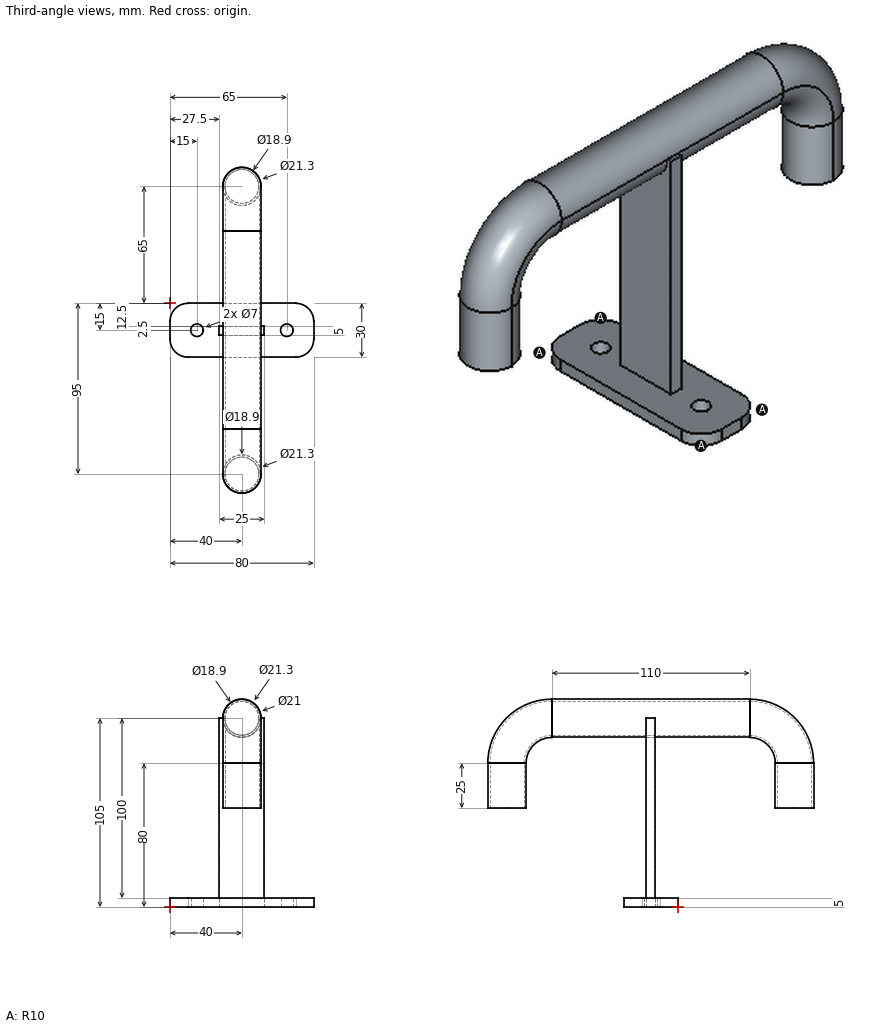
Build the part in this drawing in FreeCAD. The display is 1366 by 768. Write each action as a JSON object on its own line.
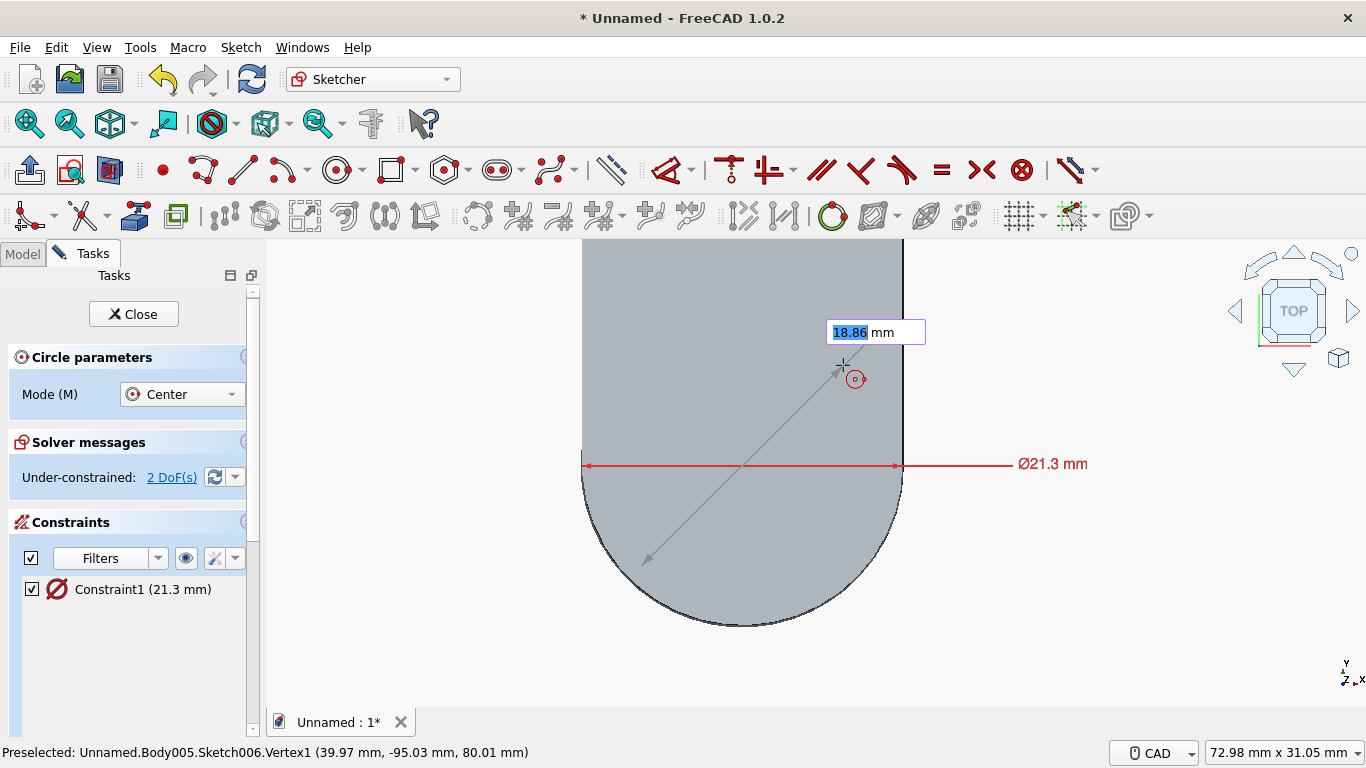
{"action": "type", "text": "18.9"}
{"action": "key", "text": "Return"}
{"action": "key", "text": "Escape"}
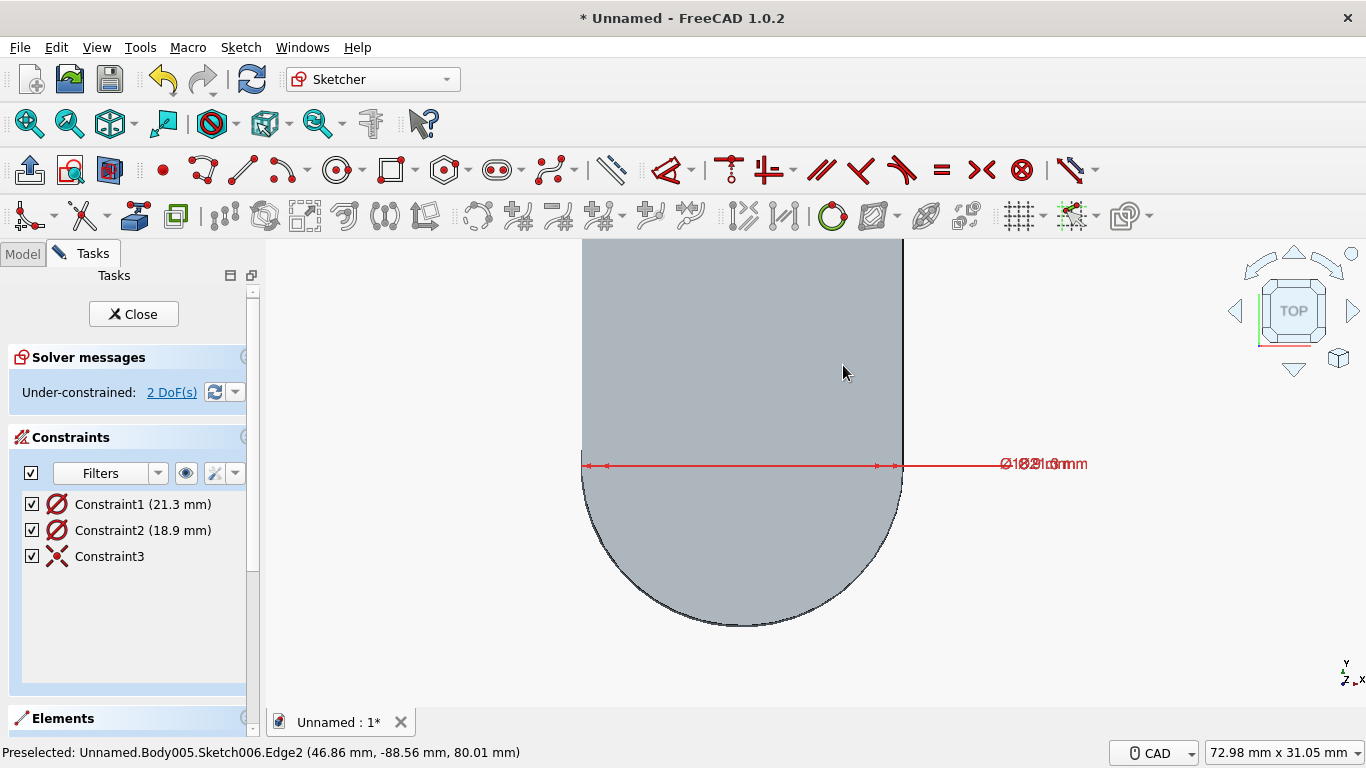
{"action": "left_click", "coordinate": [666, 170]}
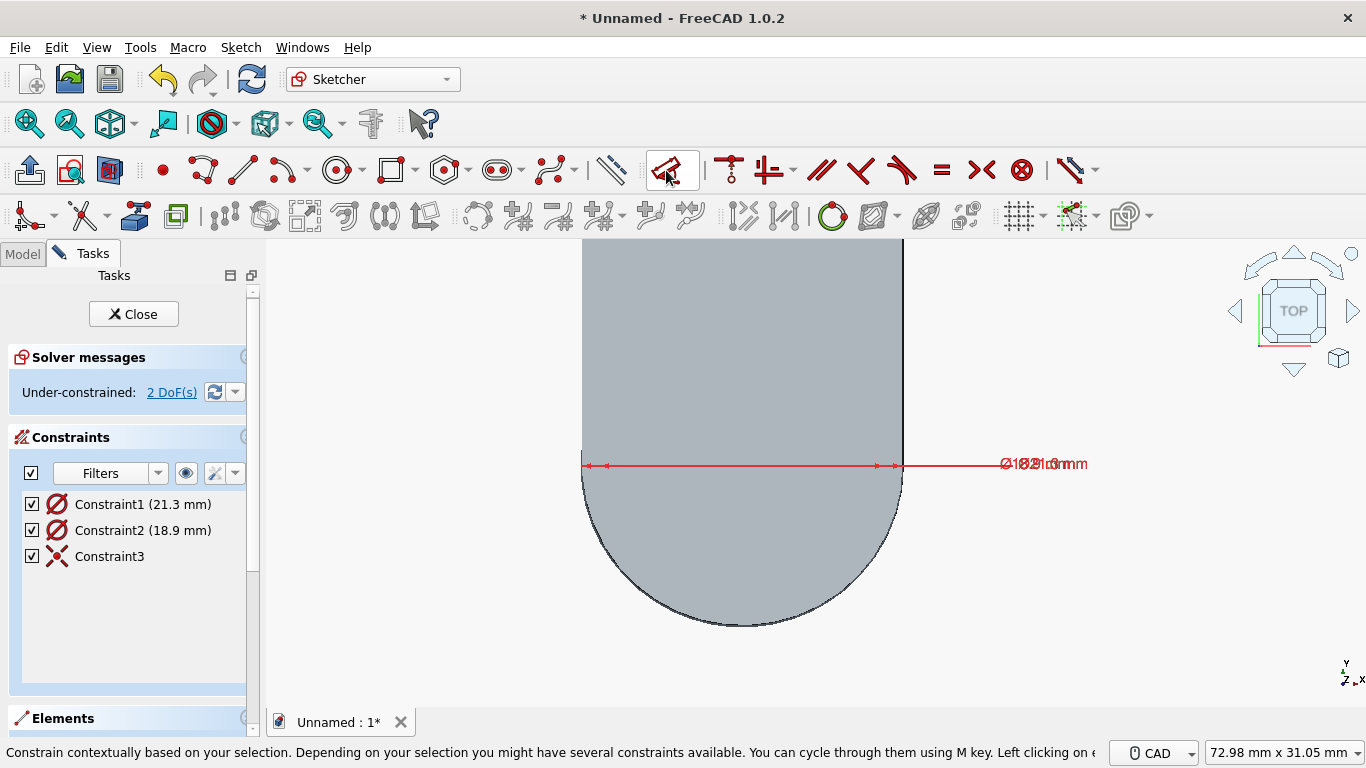
{"action": "left_click", "coordinate": [742, 466]}
{"action": "left_click", "coordinate": [518, 500]}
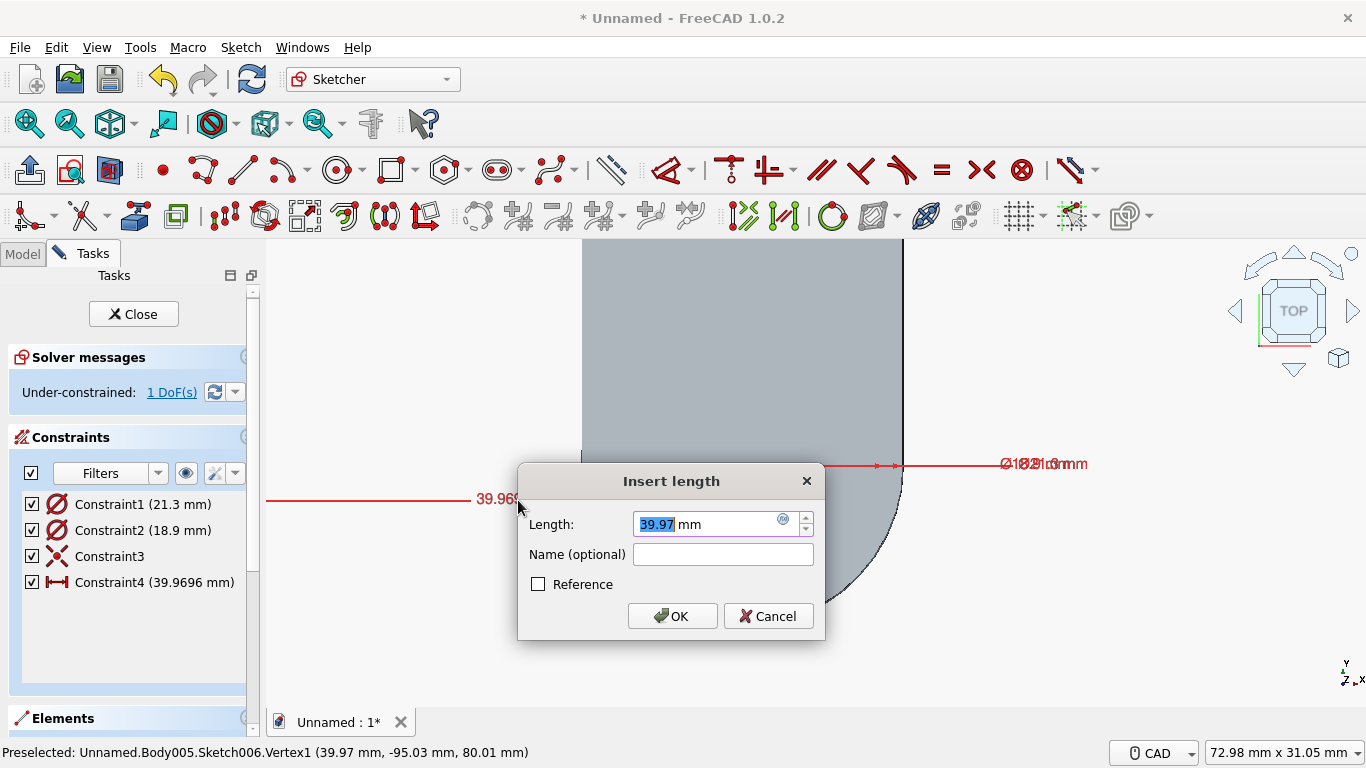
{"action": "type", "text": "40"}
{"action": "key", "text": "Return"}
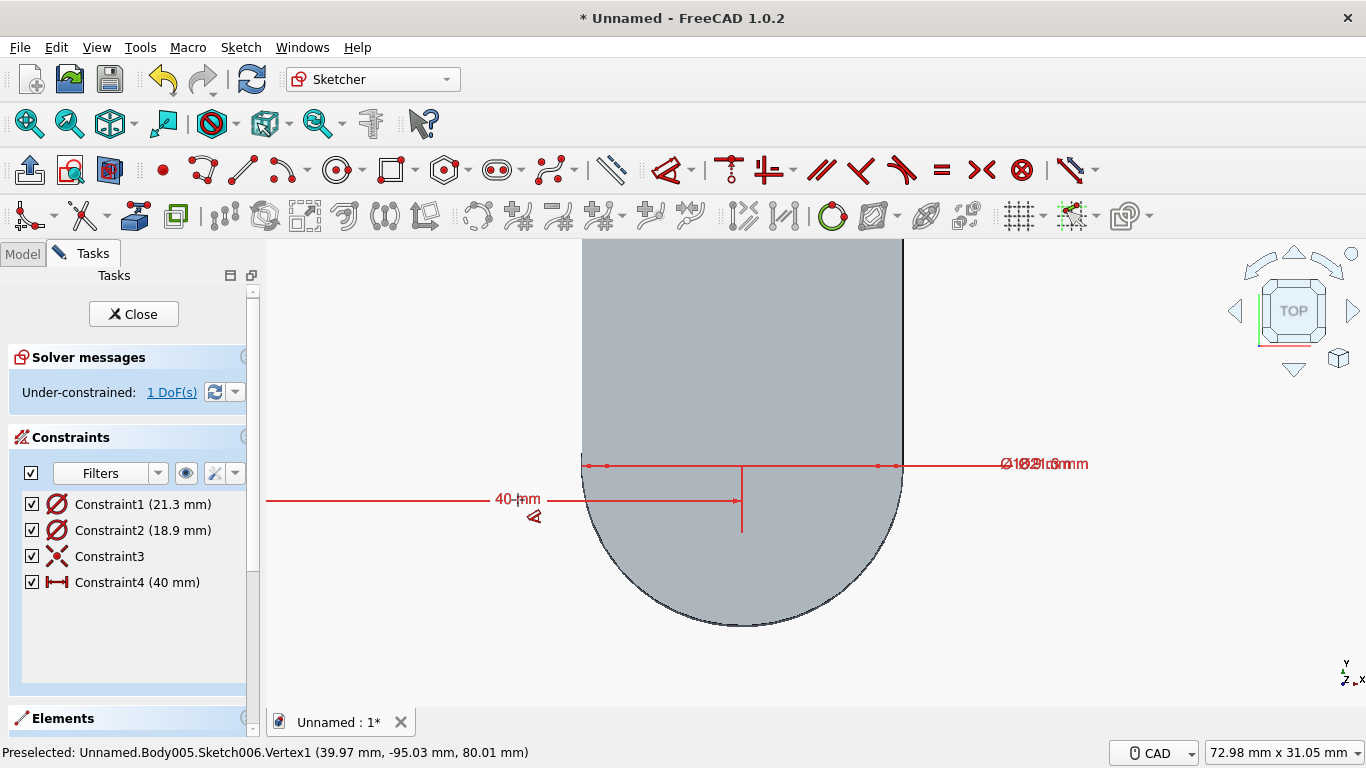
{"action": "left_click", "coordinate": [742, 466]}
{"action": "left_click", "coordinate": [776, 367]}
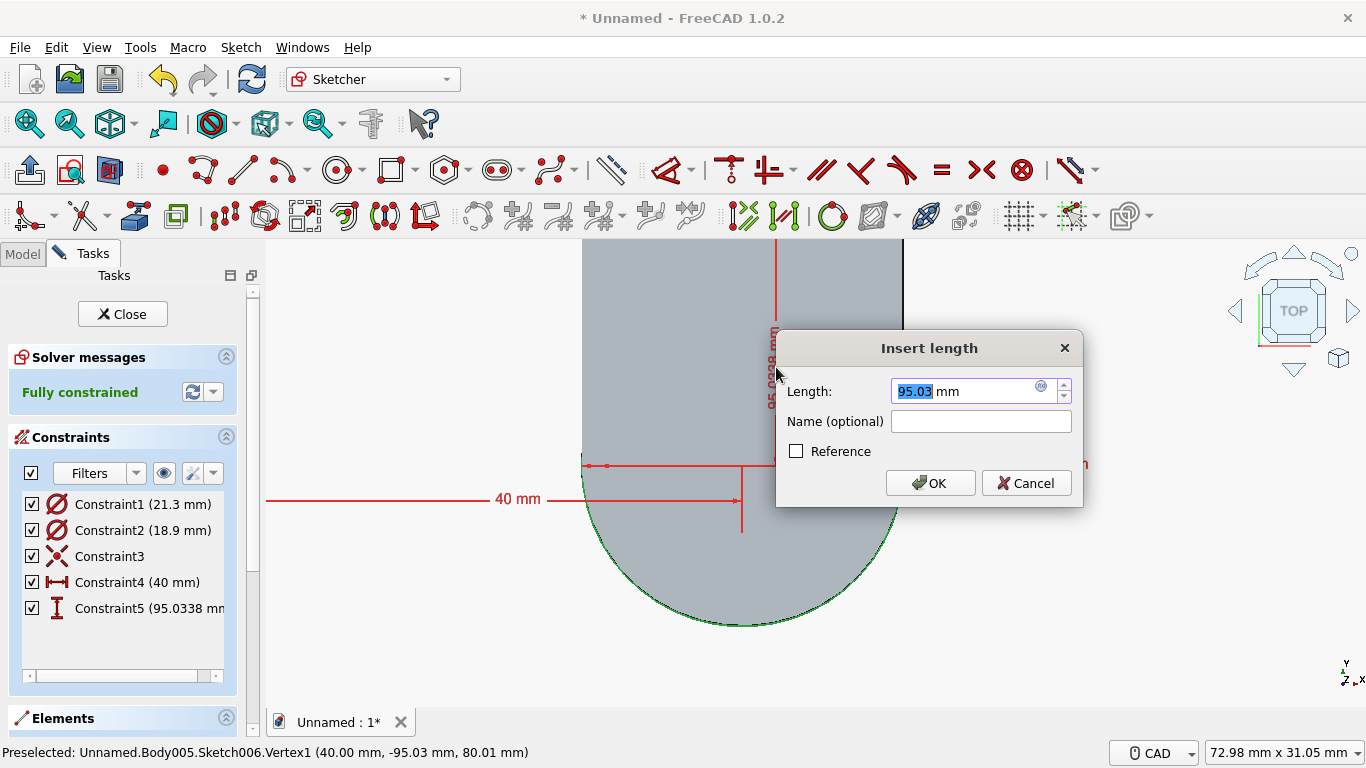
{"action": "type", "text": "95"}
{"action": "key", "text": "Return"}
{"action": "key", "text": "Escape"}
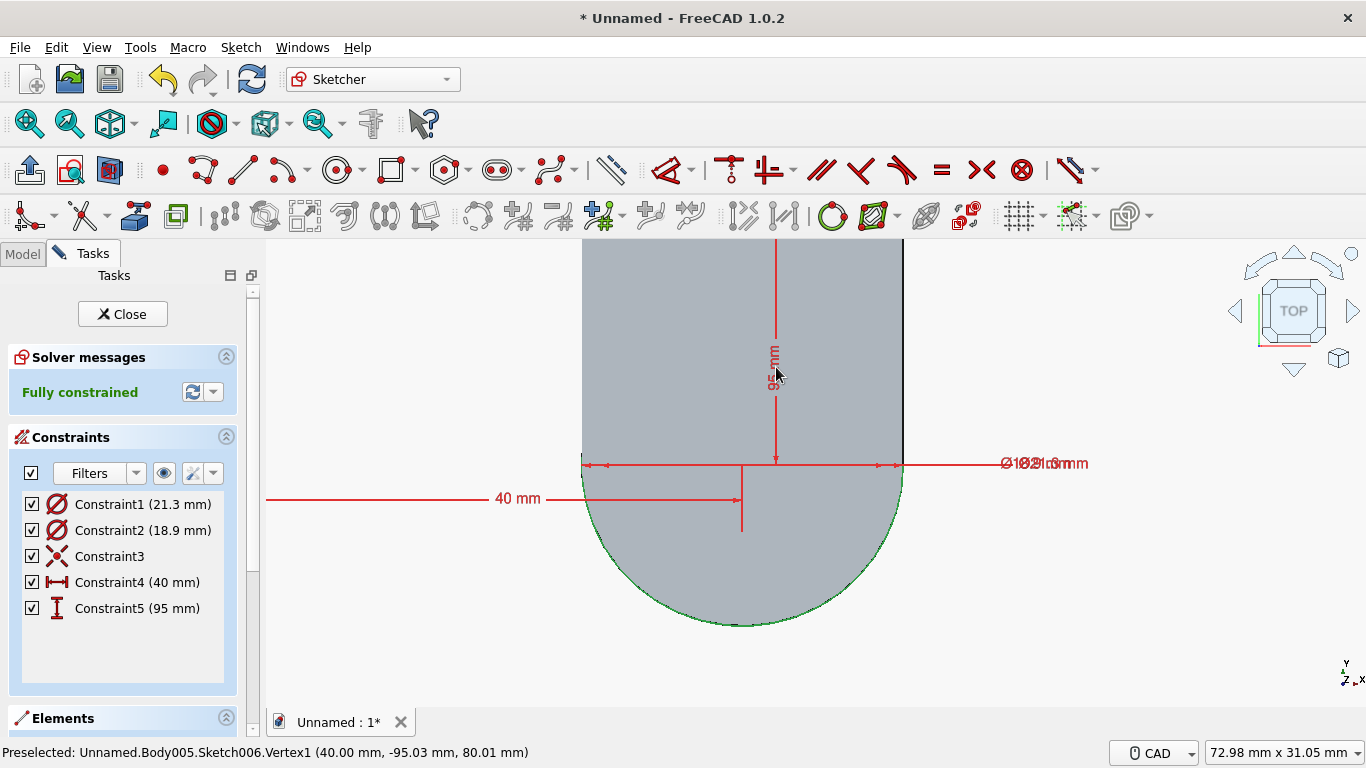
{"action": "left_click", "coordinate": [123, 314]}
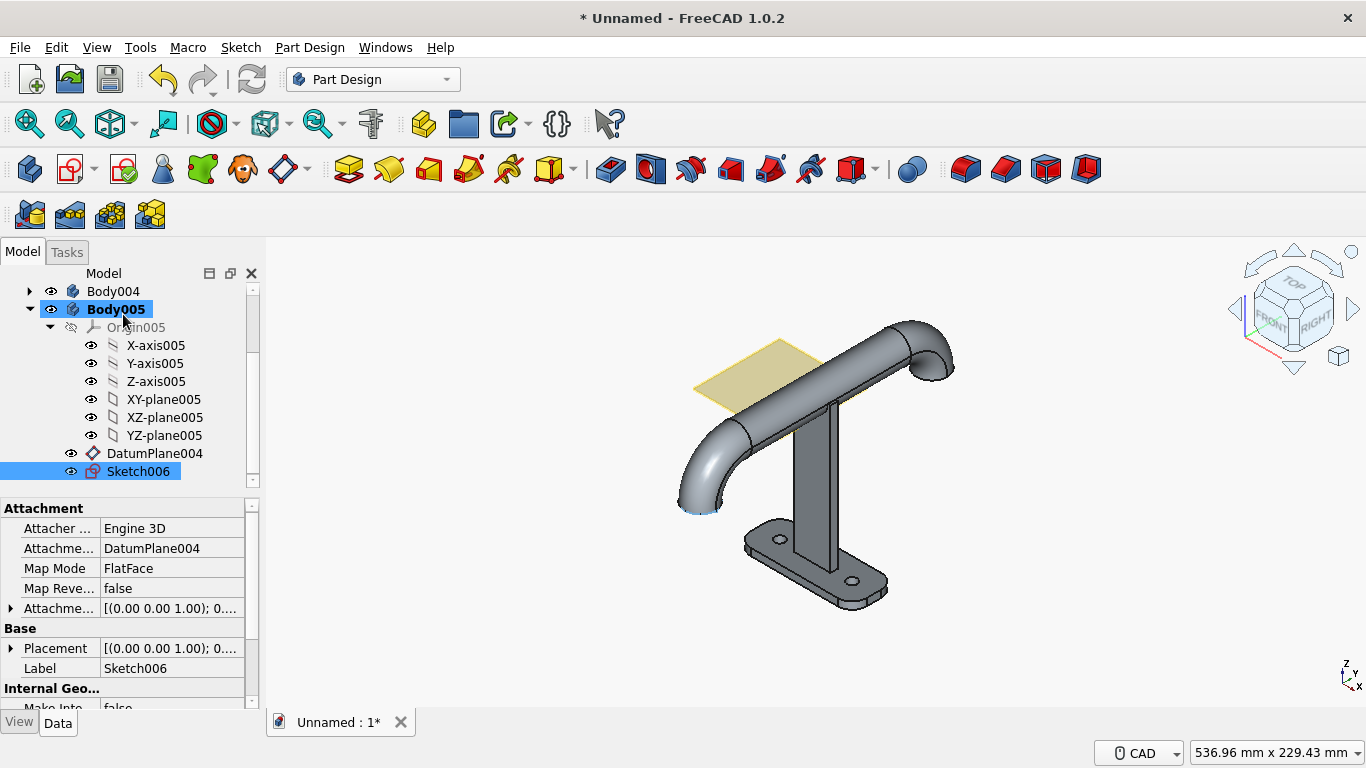
{"action": "left_click", "coordinate": [350, 170]}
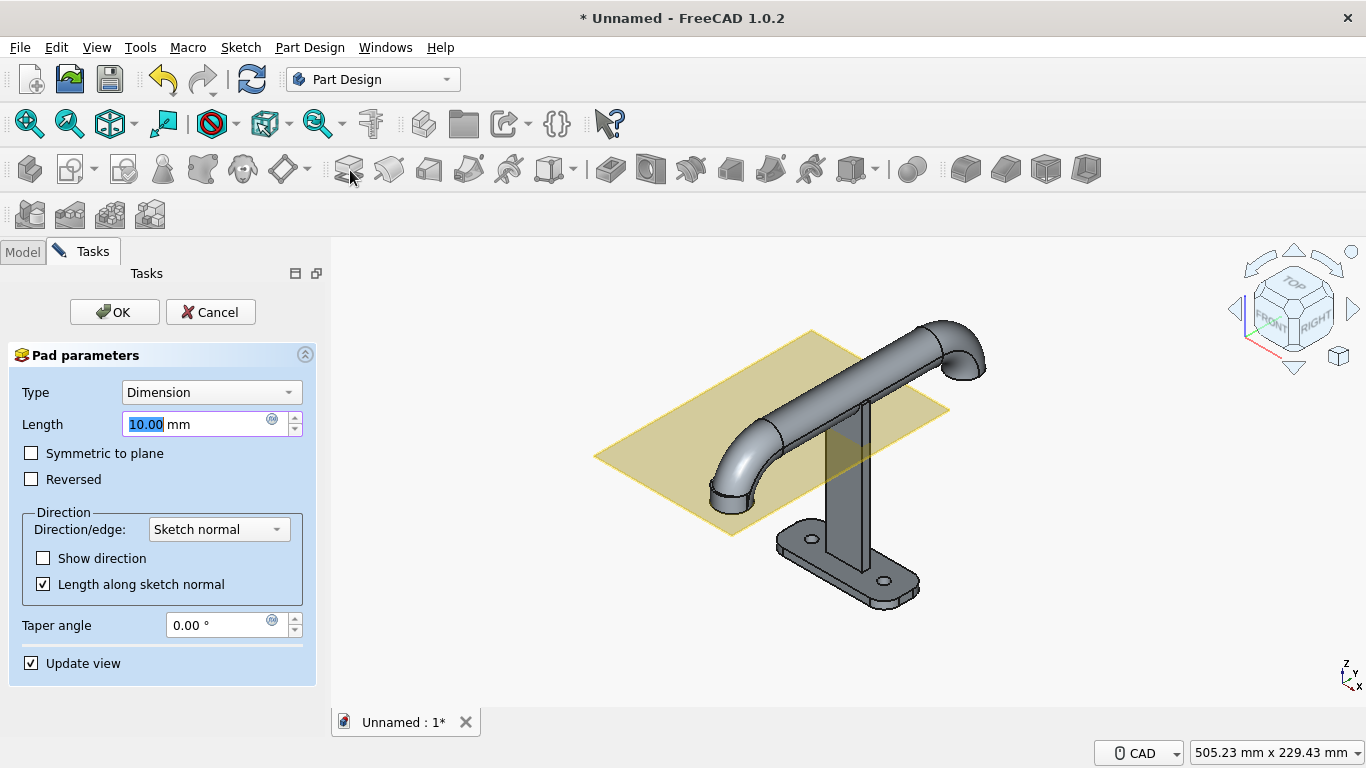
{"action": "type", "text": "25"}
{"action": "key", "text": "Tab"}